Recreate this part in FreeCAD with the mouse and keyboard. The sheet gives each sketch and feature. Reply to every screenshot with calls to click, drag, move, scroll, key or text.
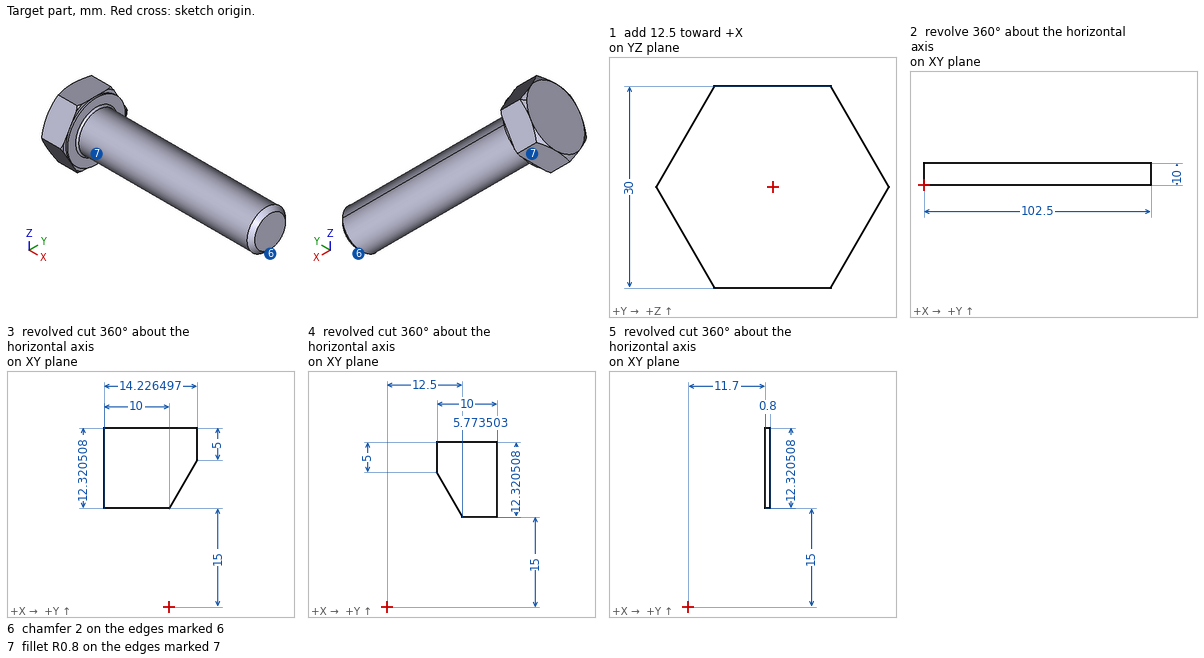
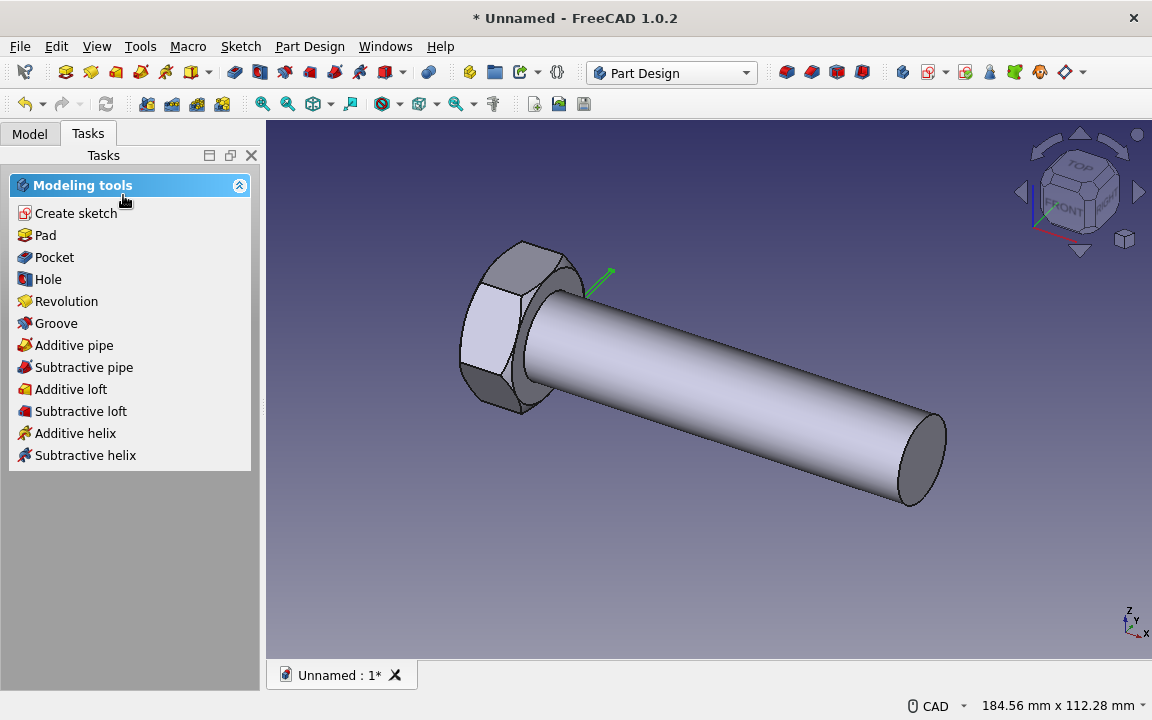
click(285, 72)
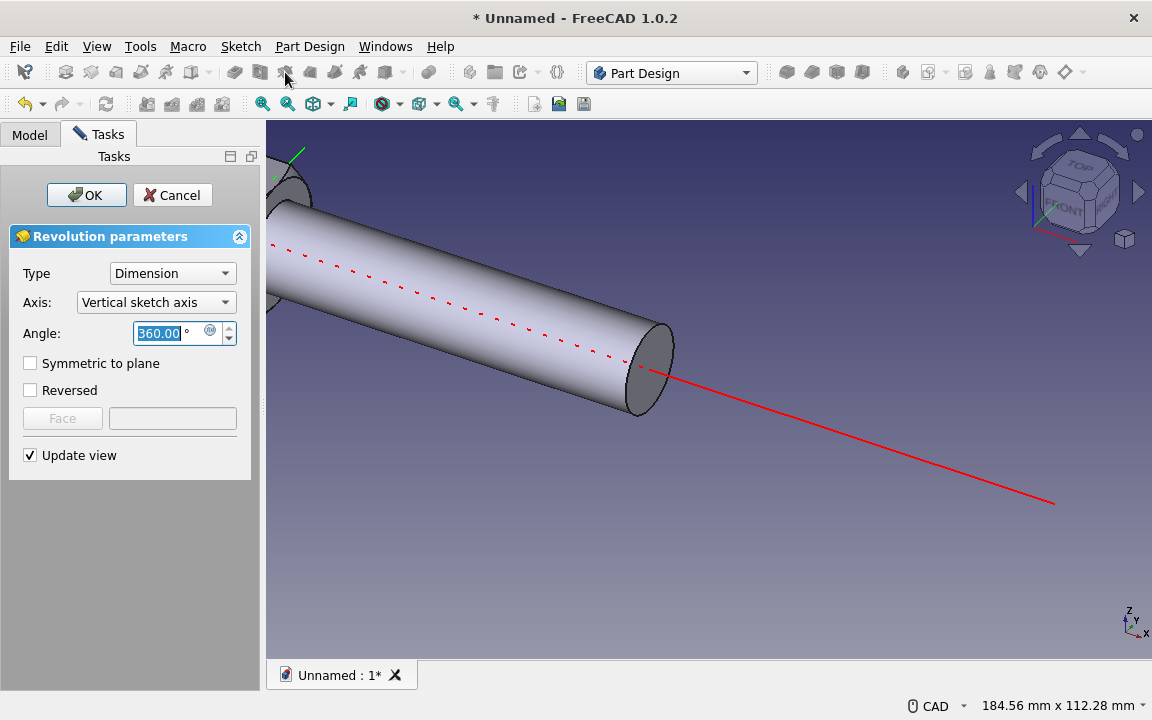
click(157, 302)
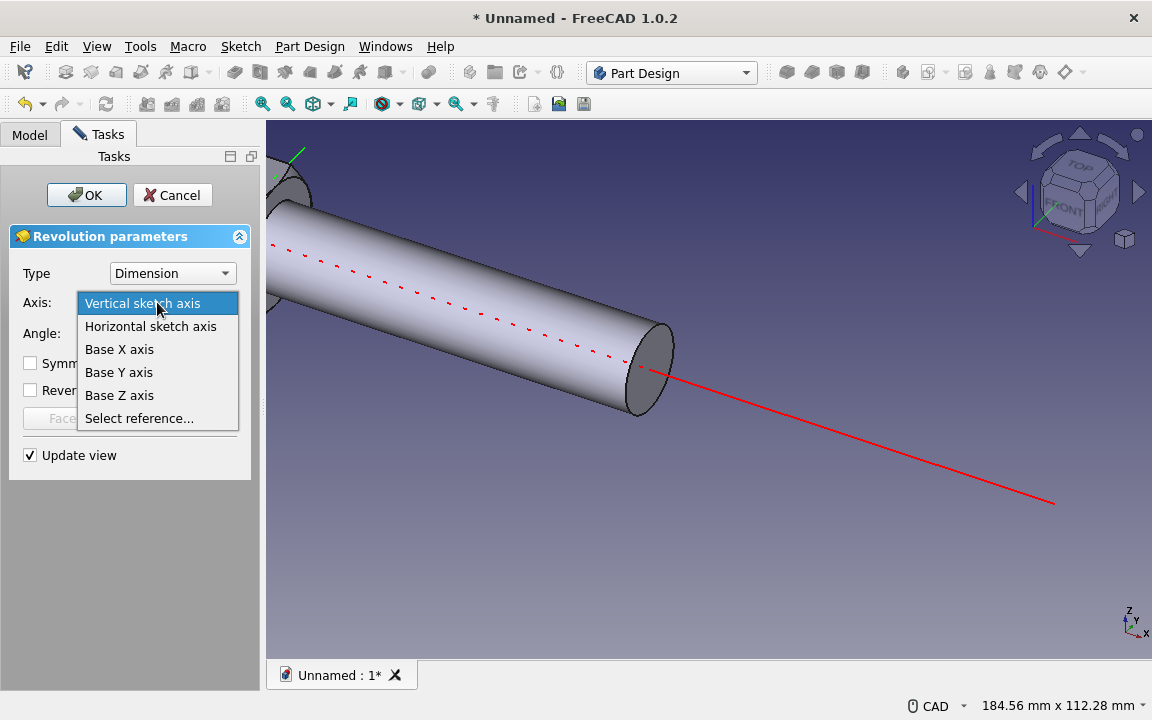
click(156, 326)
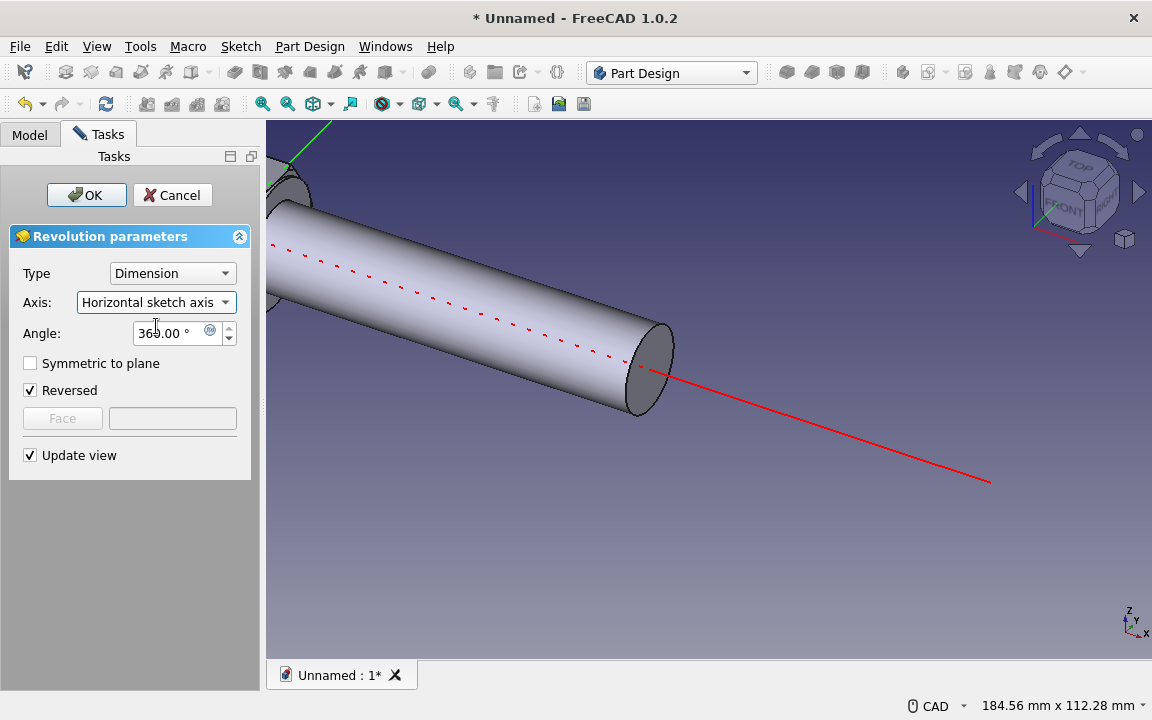
click(87, 195)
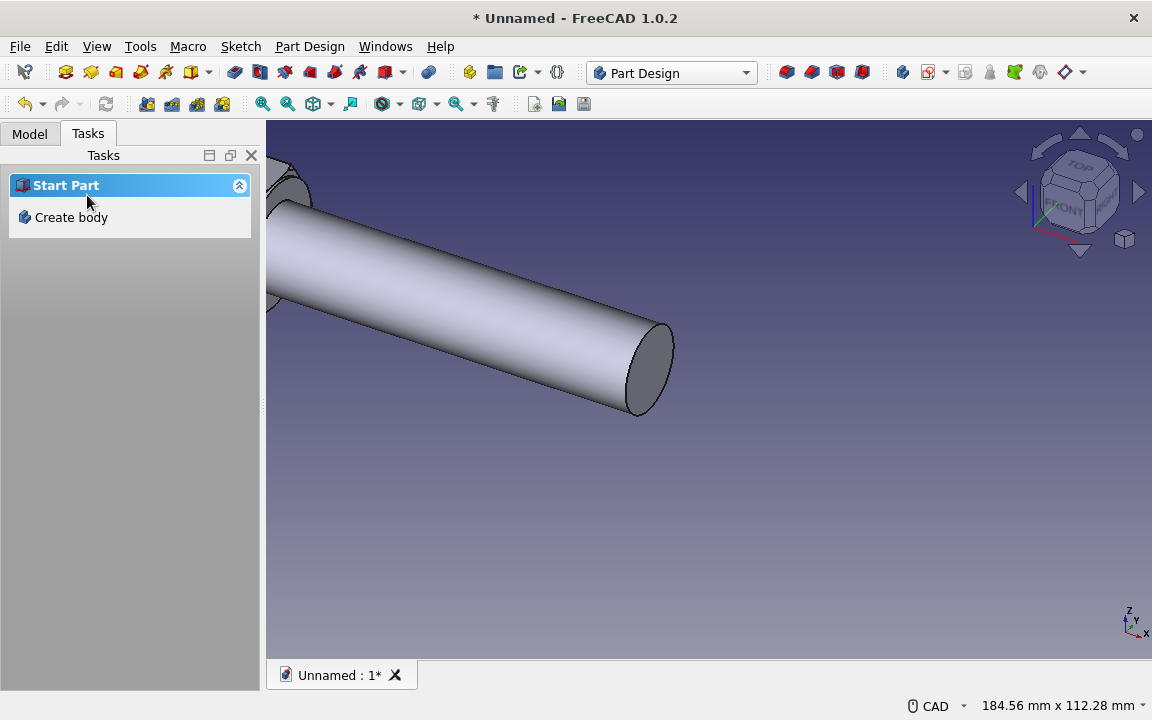
click(263, 104)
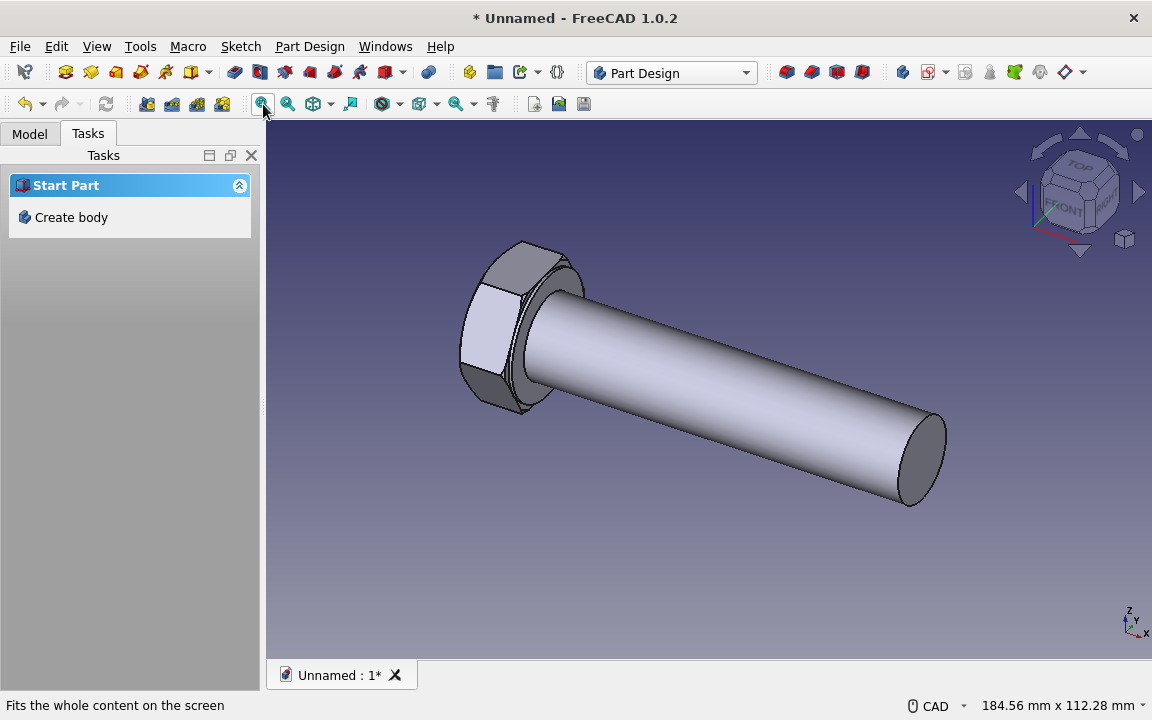
click(898, 483)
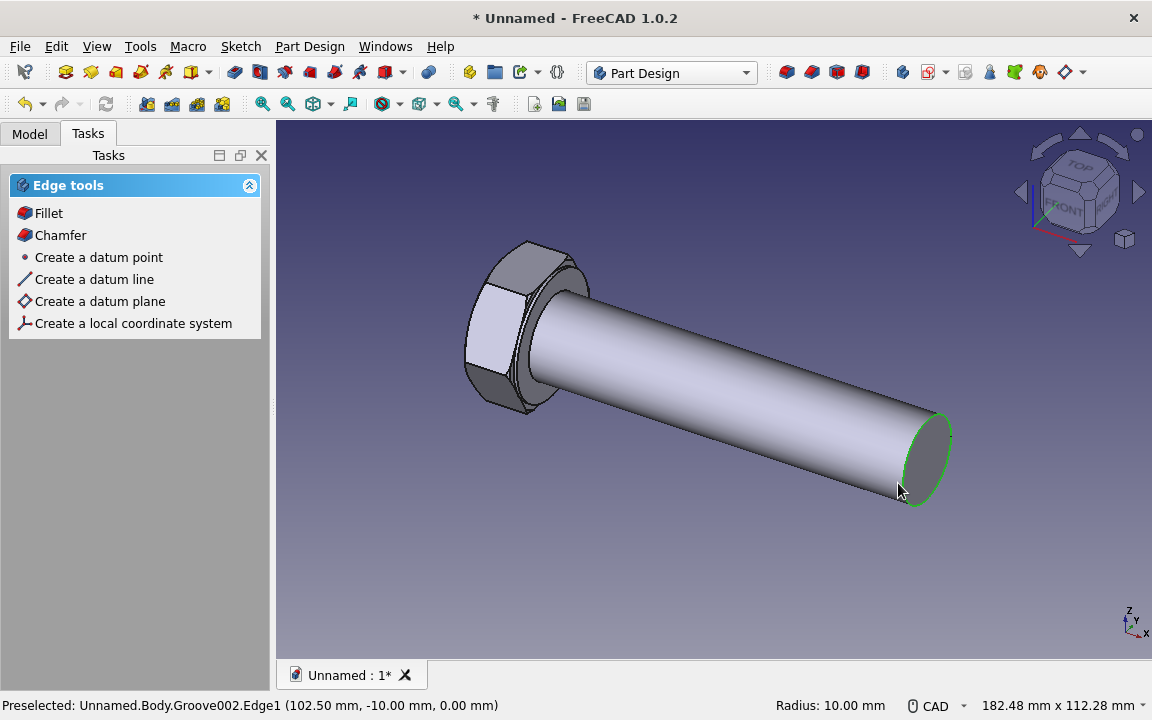
click(812, 72)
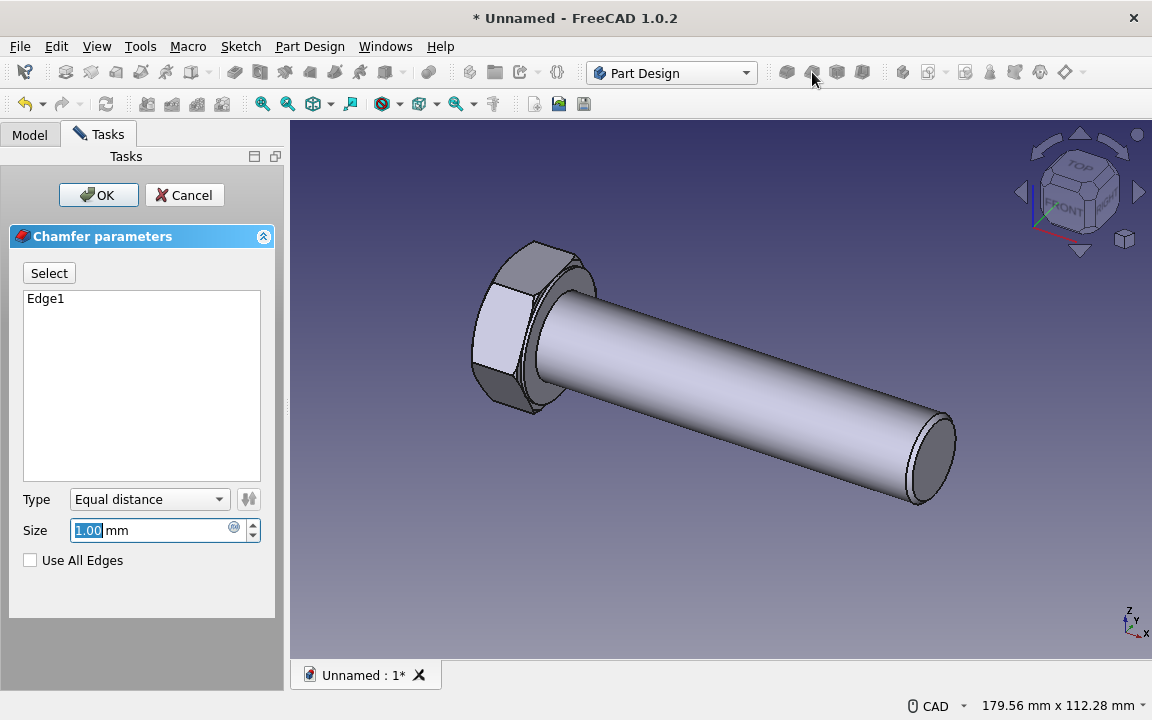
text(2)
key(Tab)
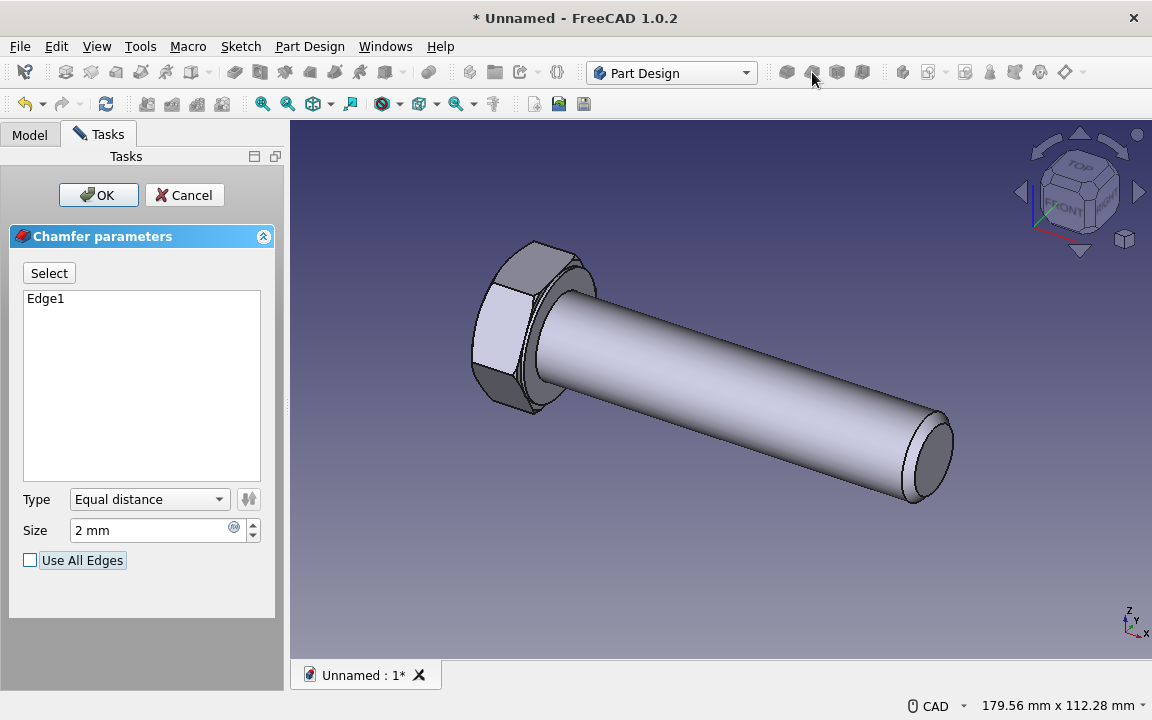
click(99, 195)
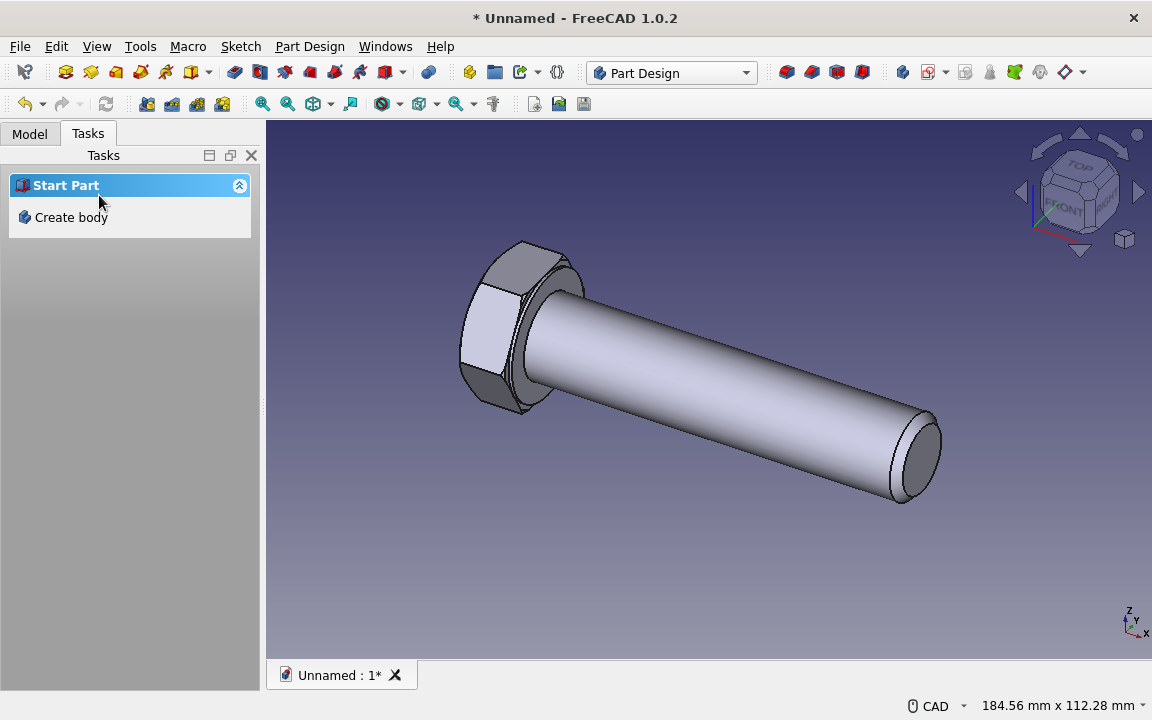
key(0)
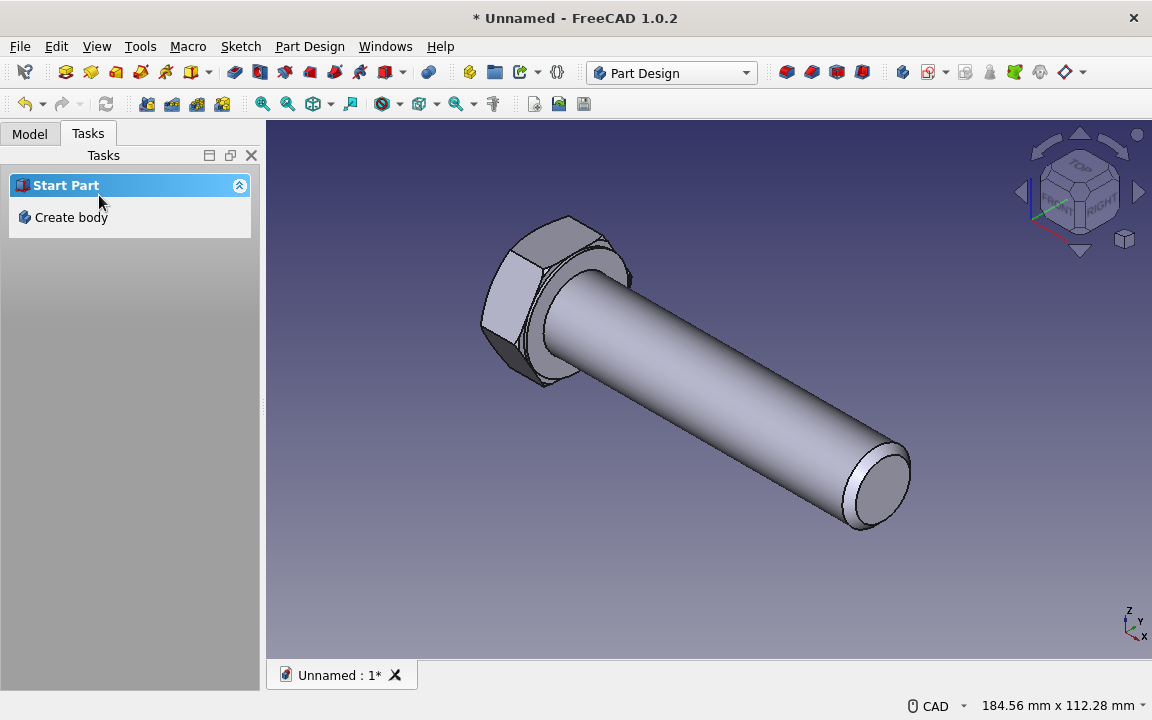
key(2)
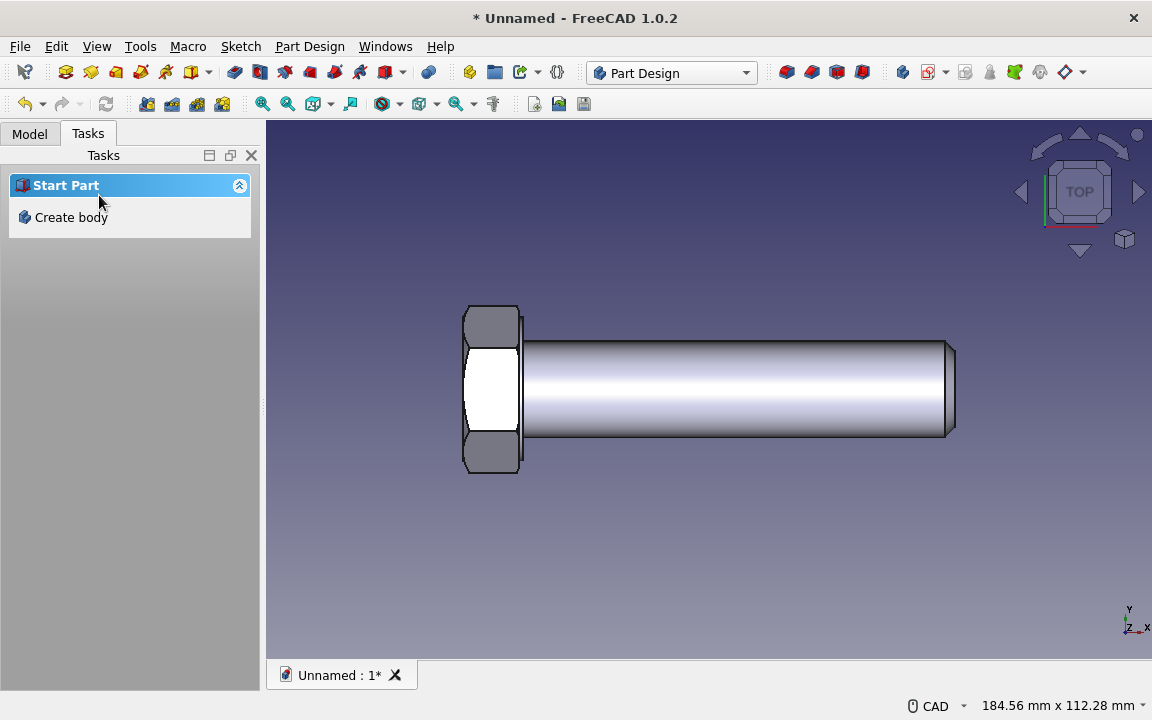
key(1)